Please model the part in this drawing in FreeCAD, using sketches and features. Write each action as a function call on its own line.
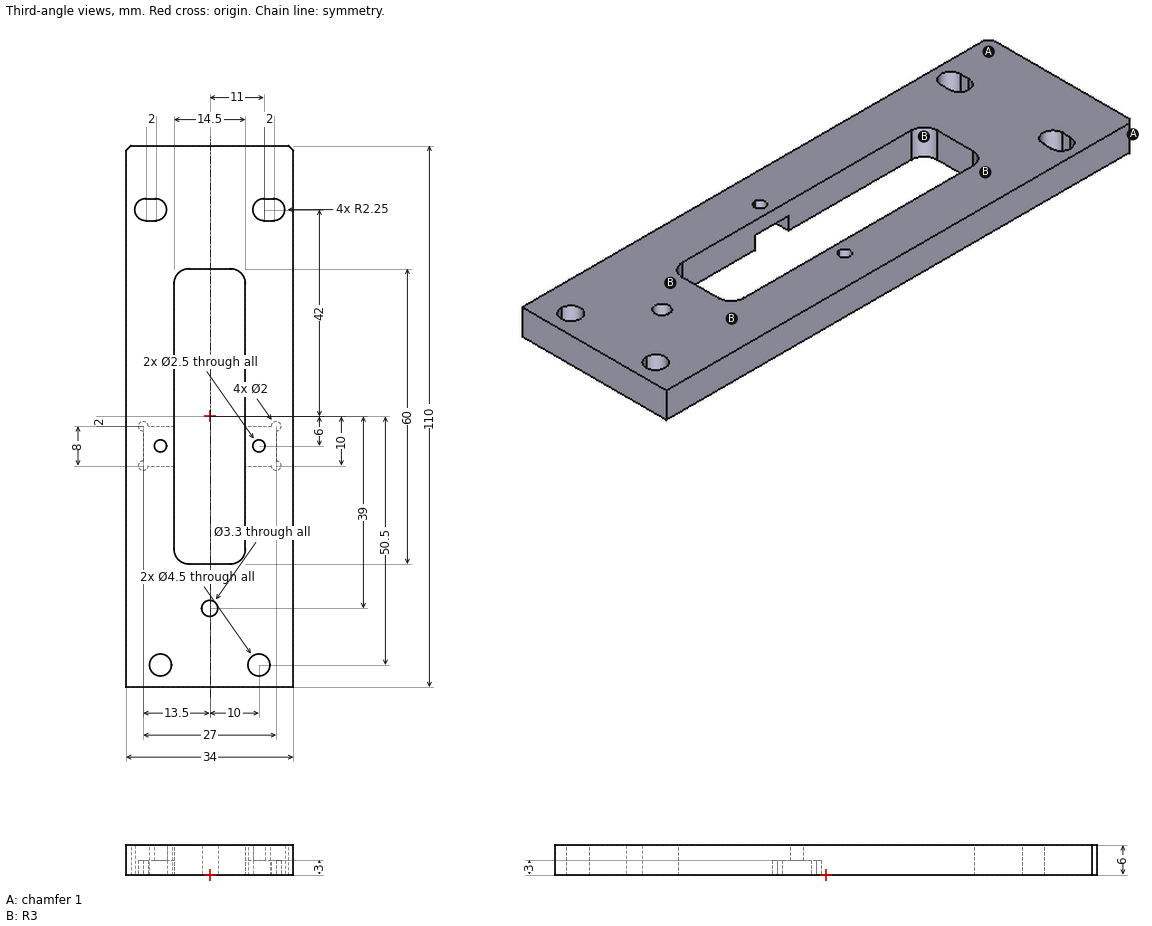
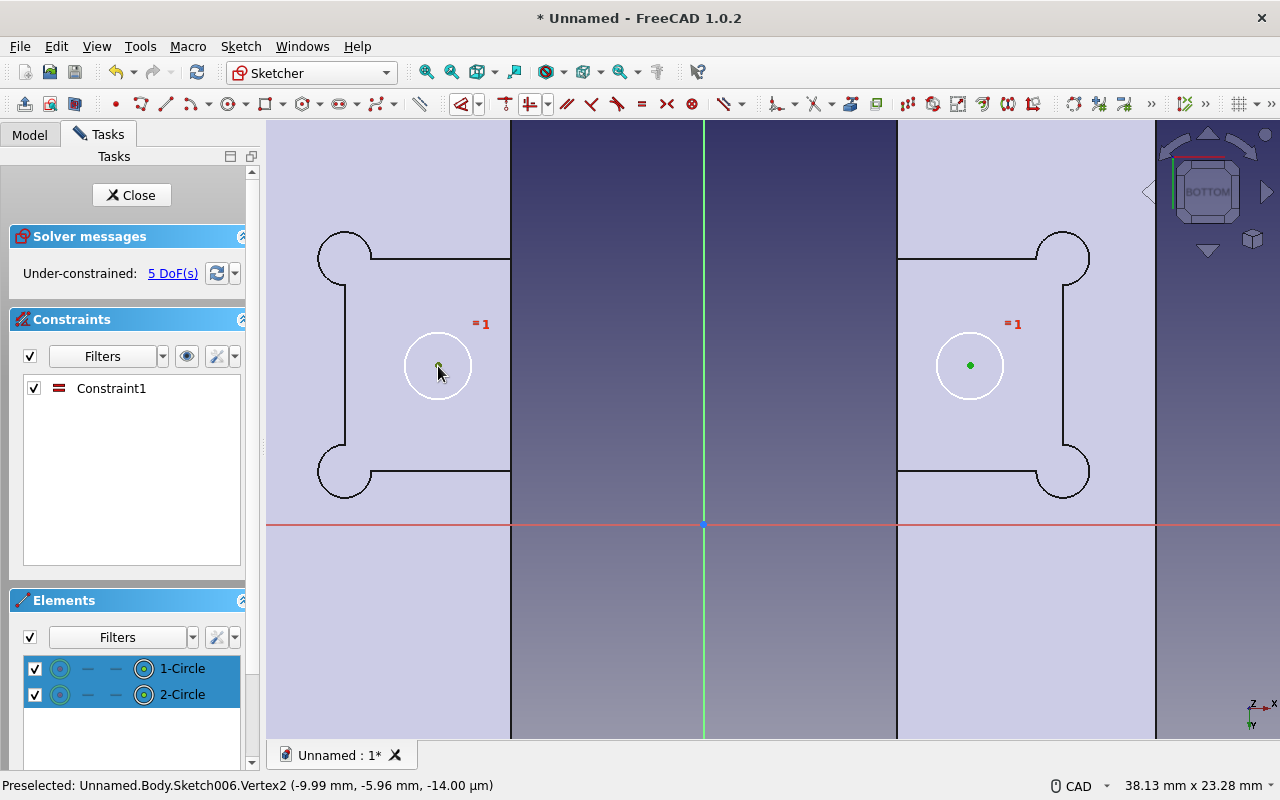
click(704, 671)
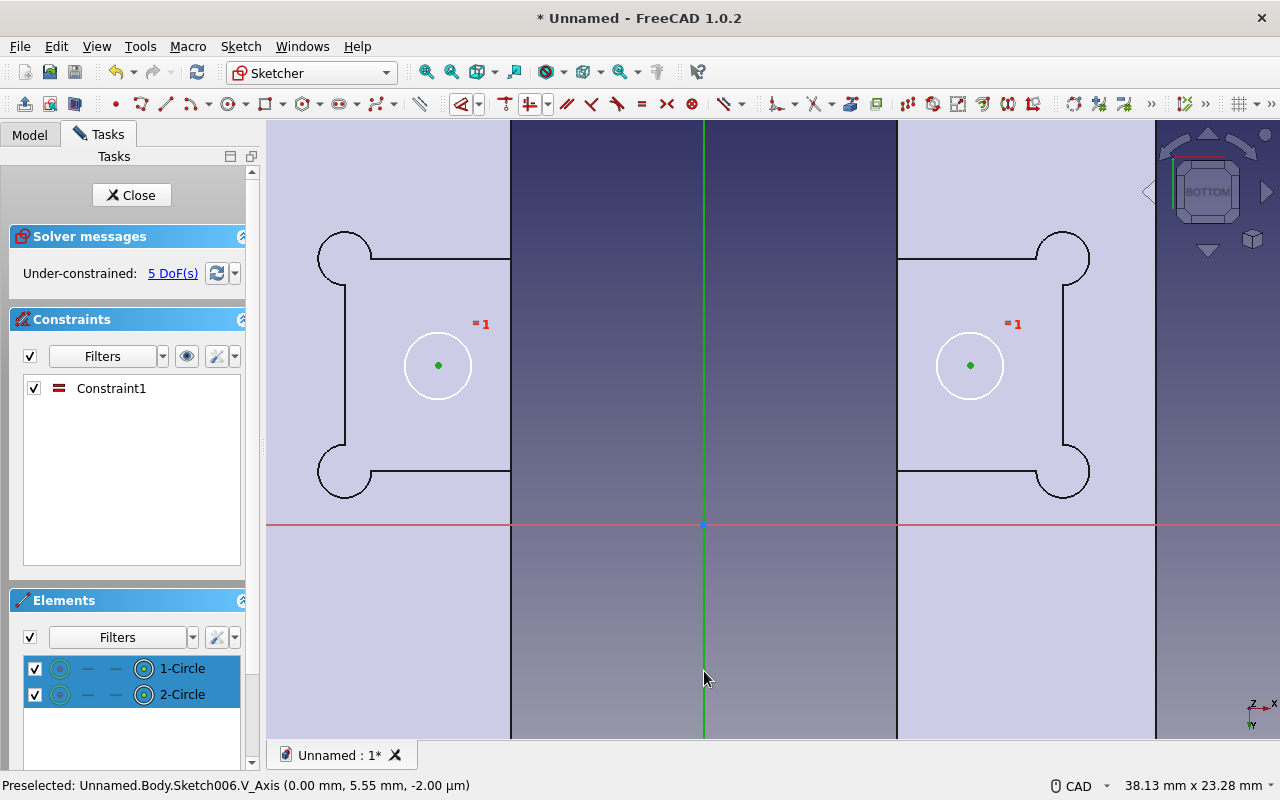
key(s)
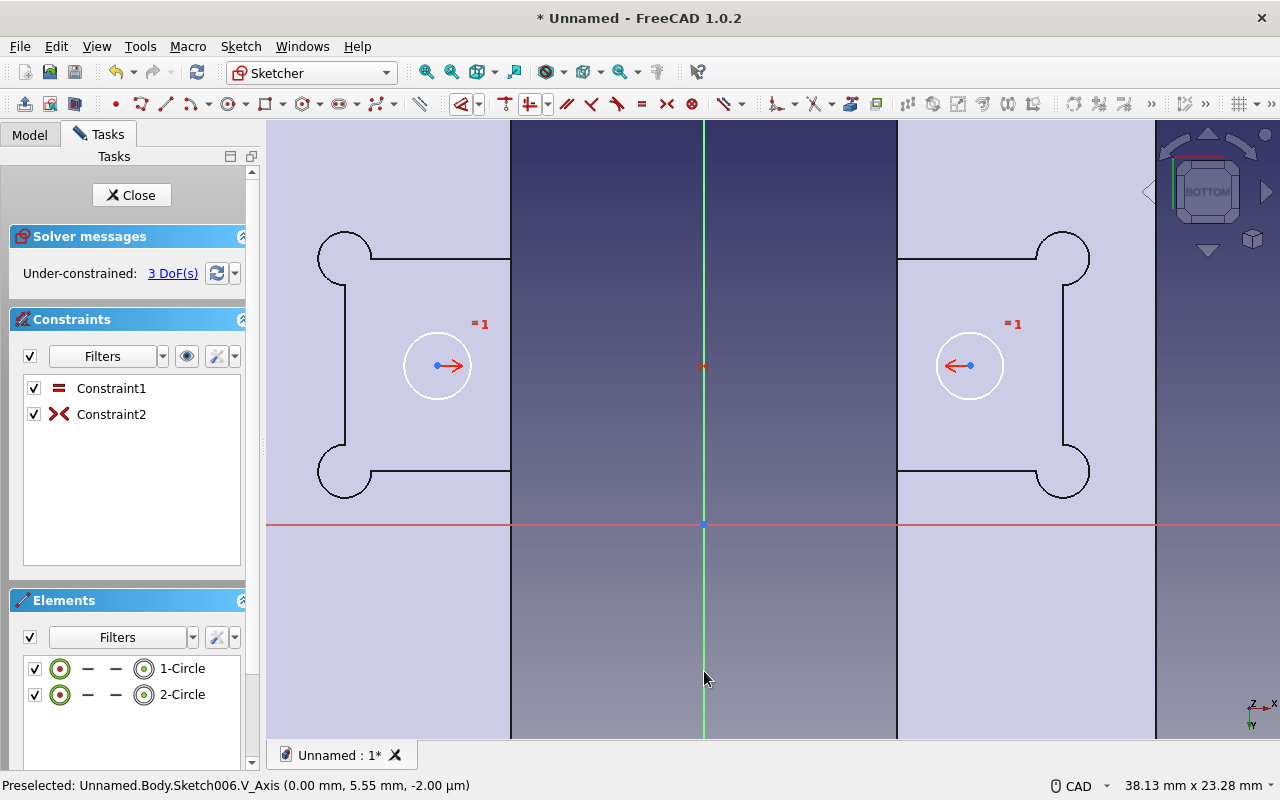
click(993, 342)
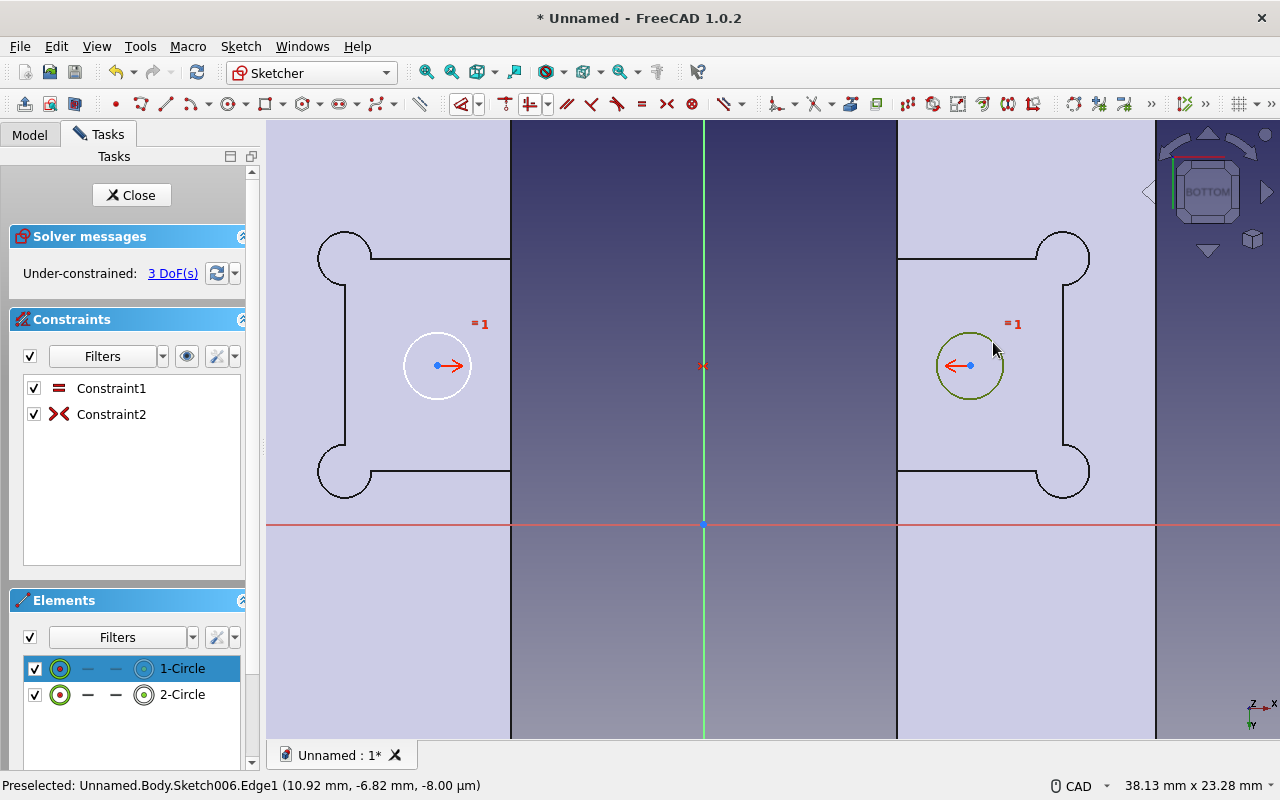
key(k)
key(o)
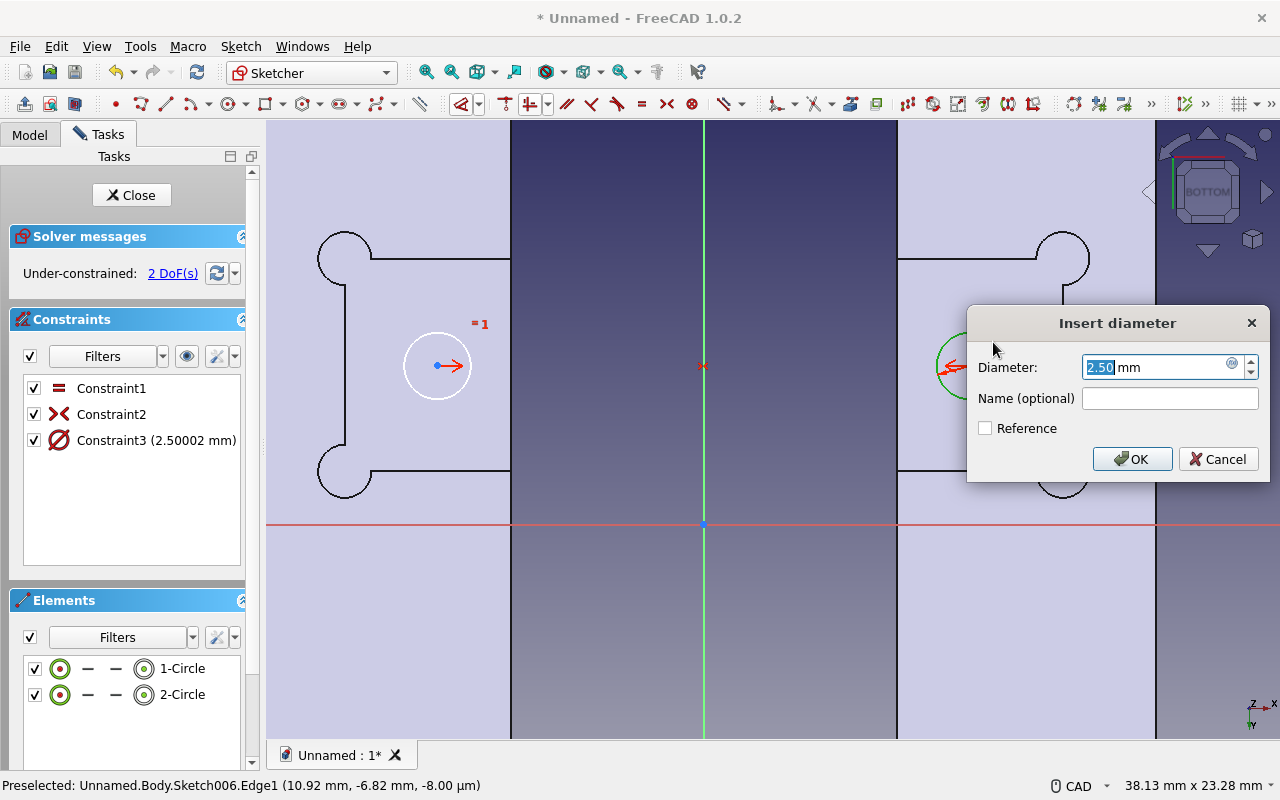
text(2.5)
key(Return)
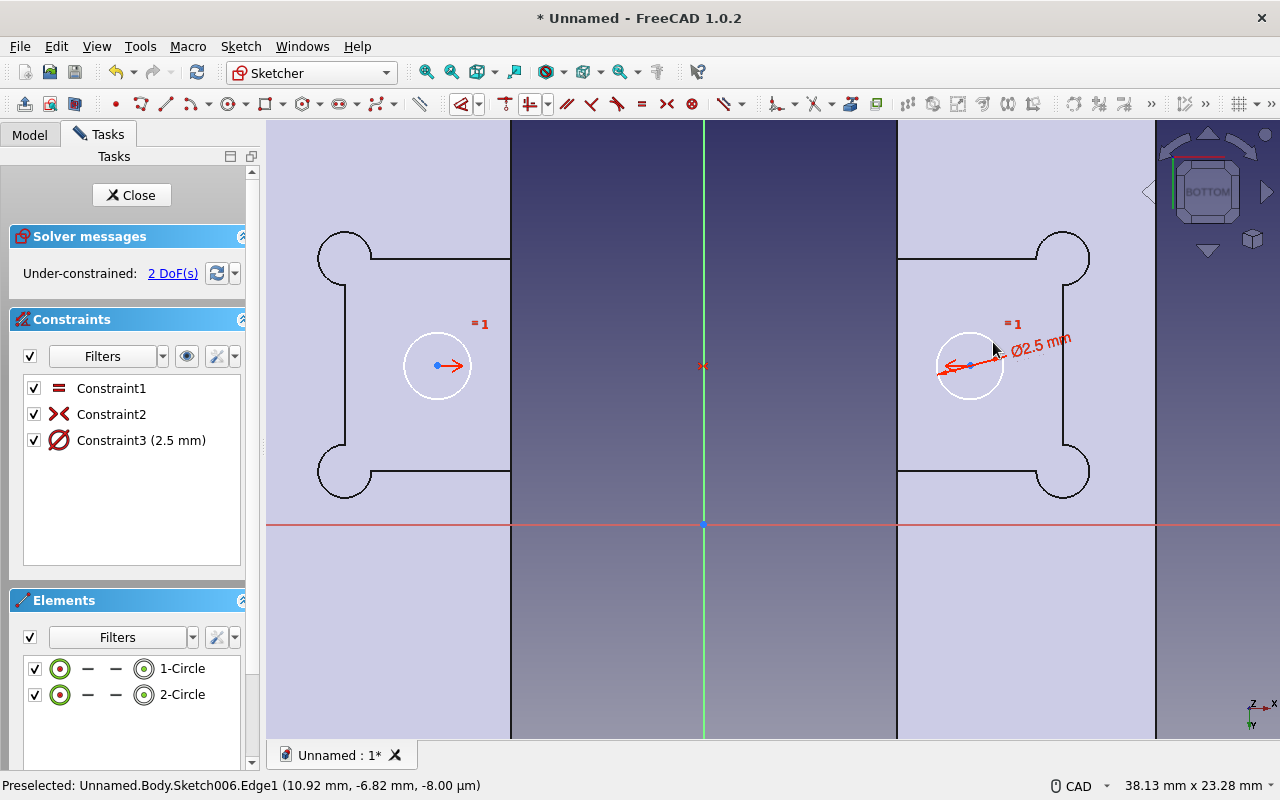
click(970, 366)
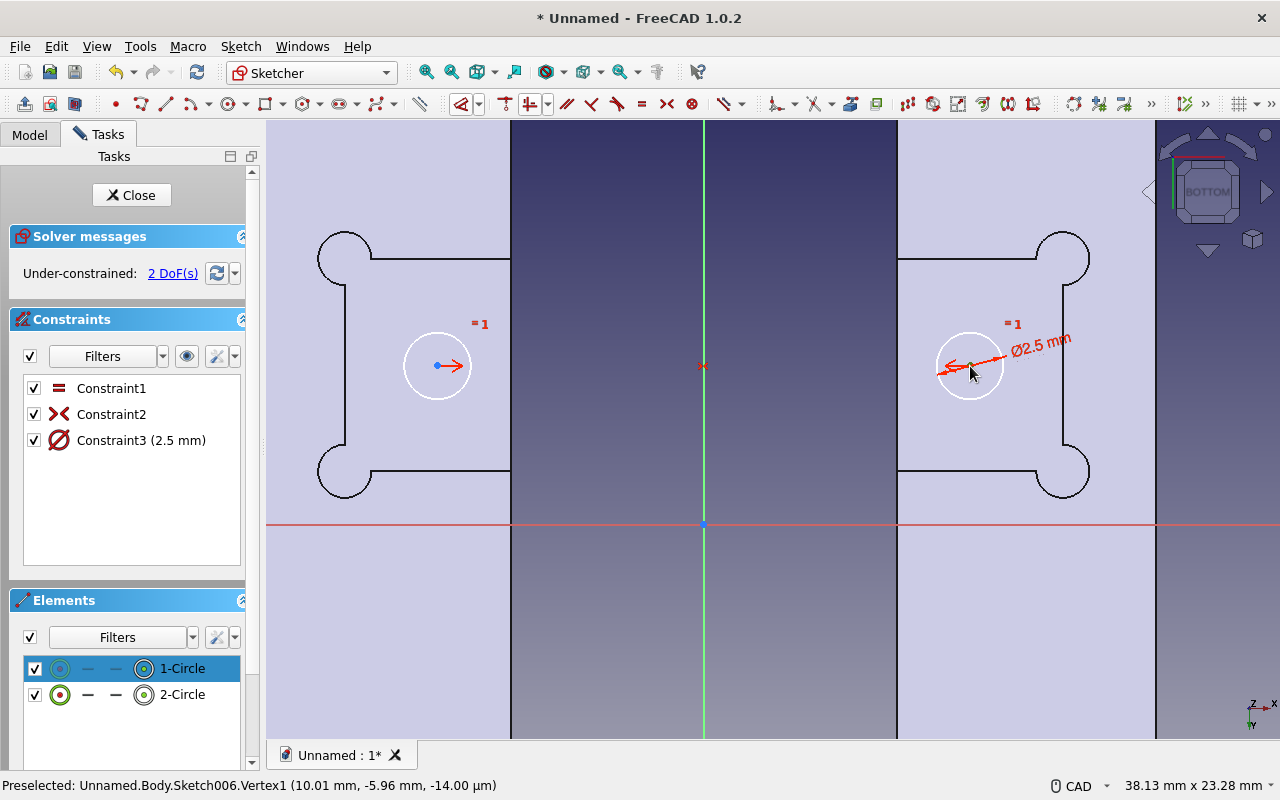
key(i)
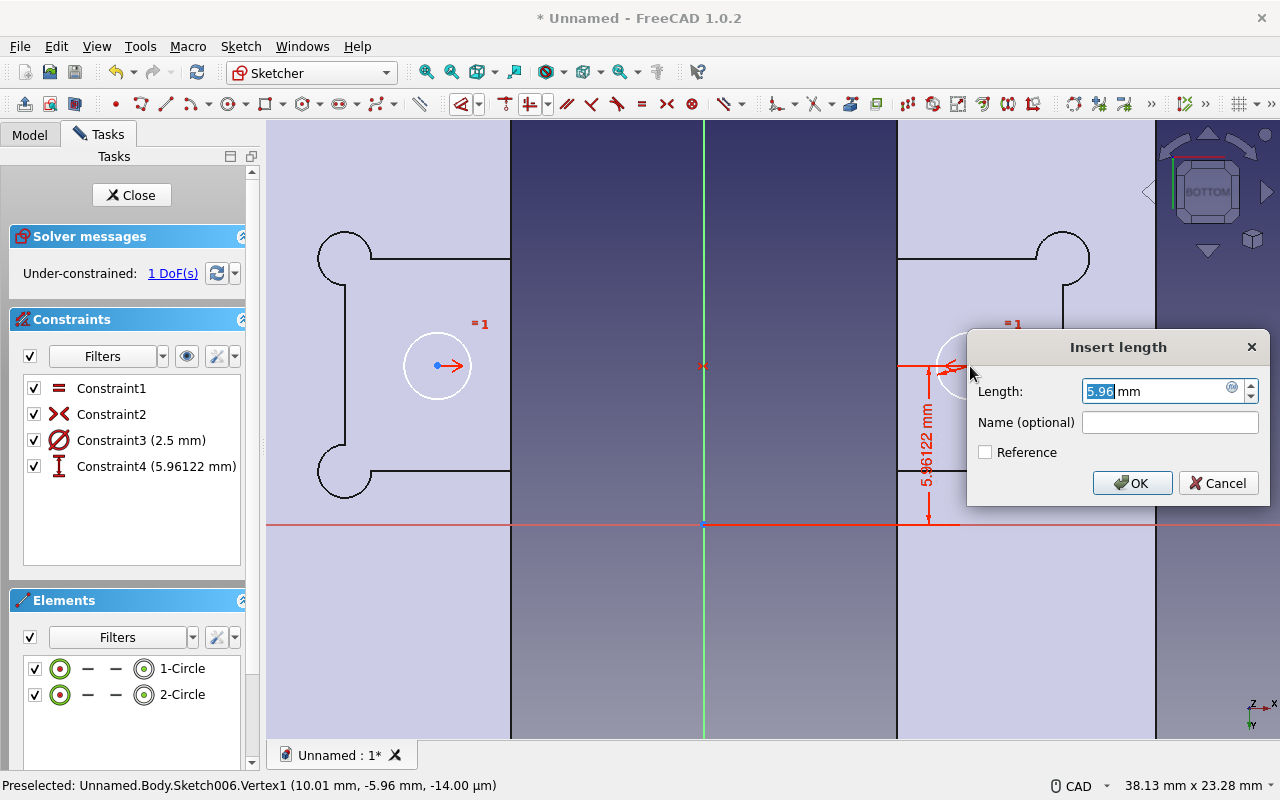
text(6)
key(Return)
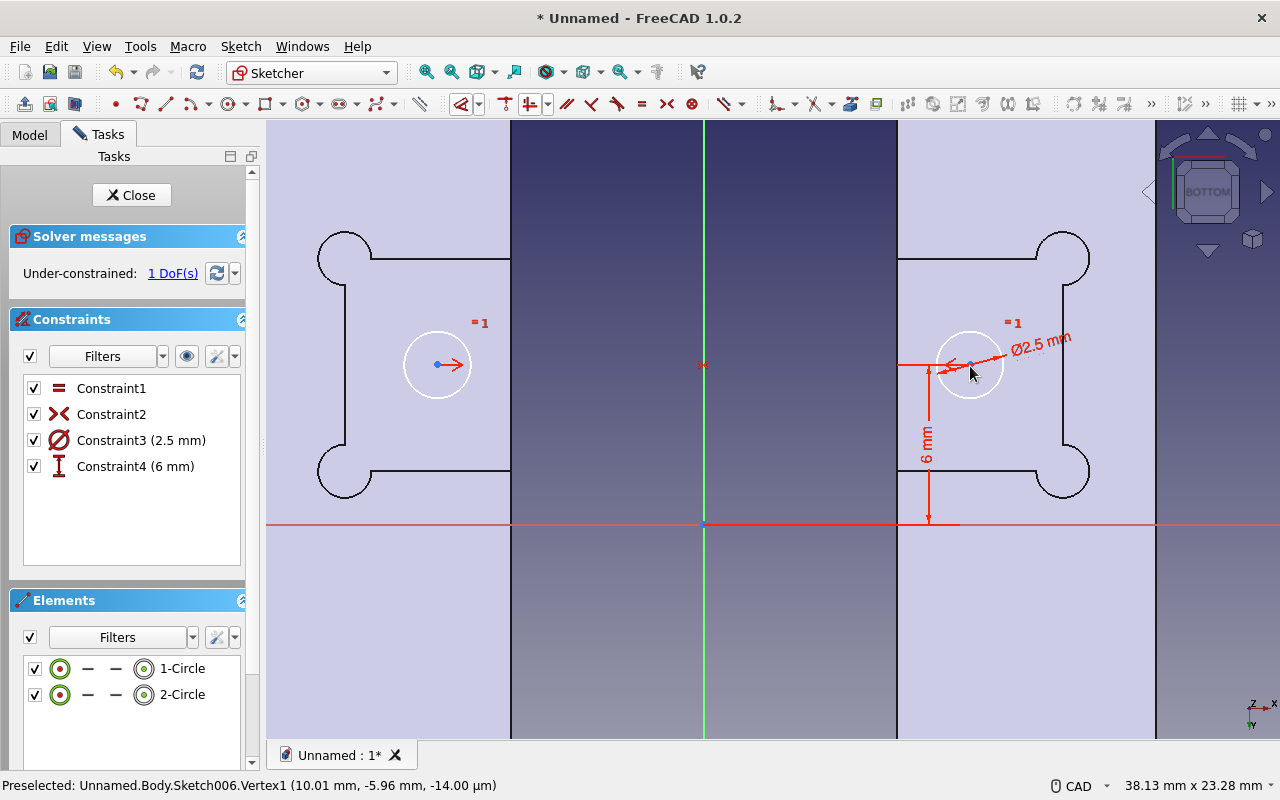
click(970, 365)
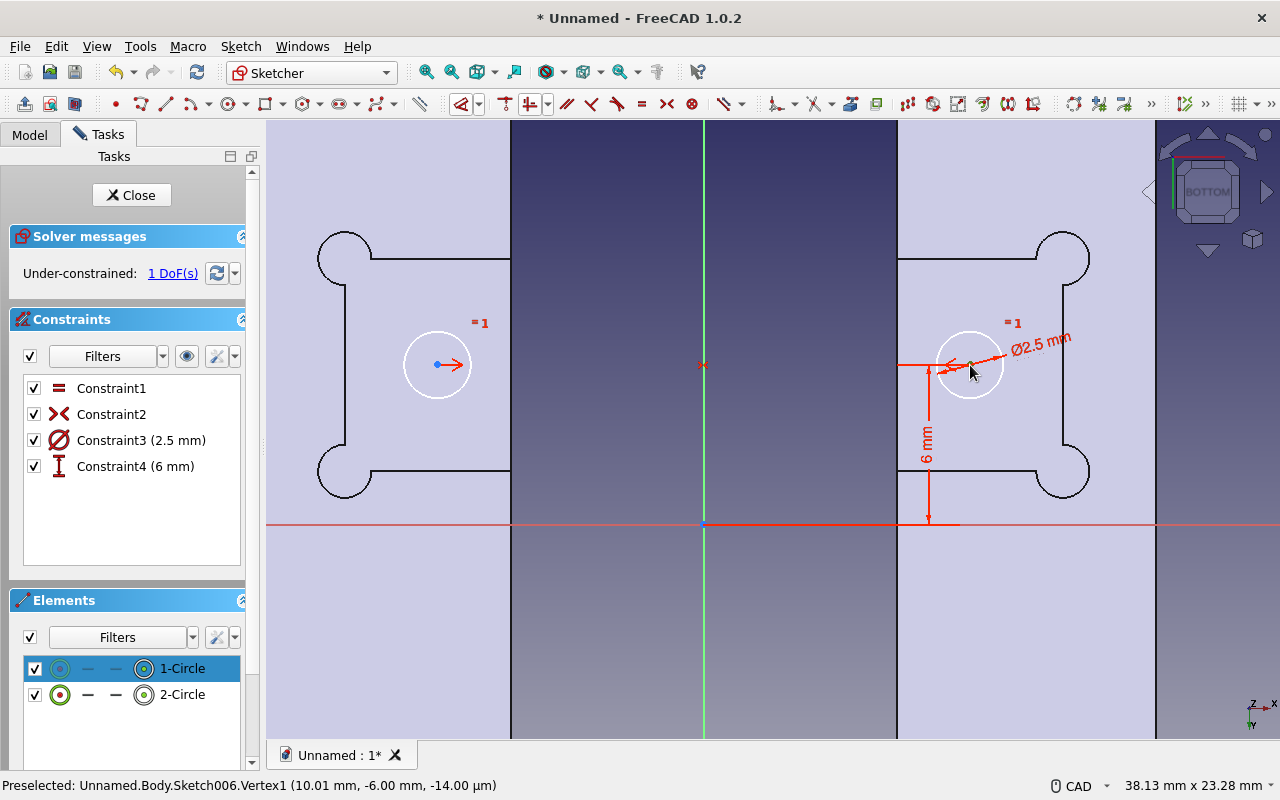
key(l)